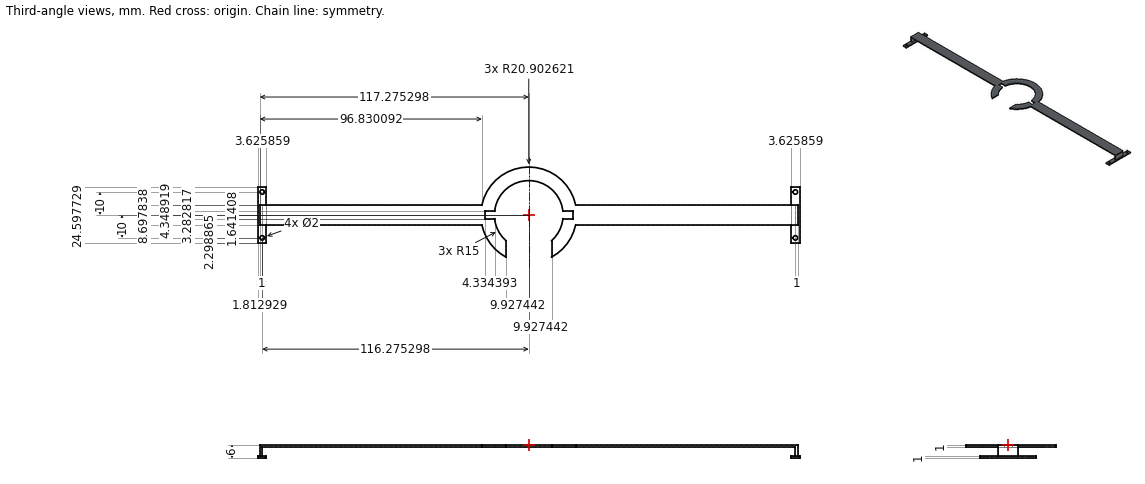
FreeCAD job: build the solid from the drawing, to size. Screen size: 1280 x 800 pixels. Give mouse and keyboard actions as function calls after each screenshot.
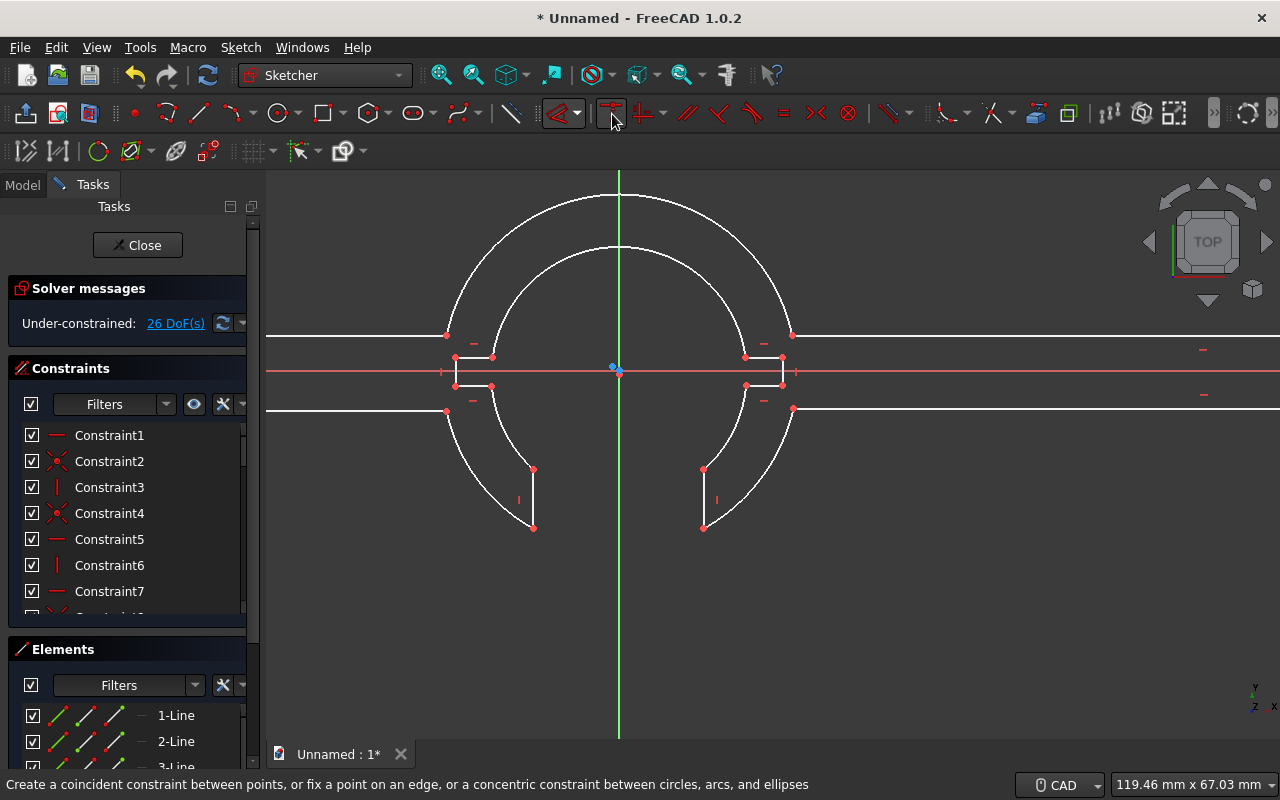
click(462, 454)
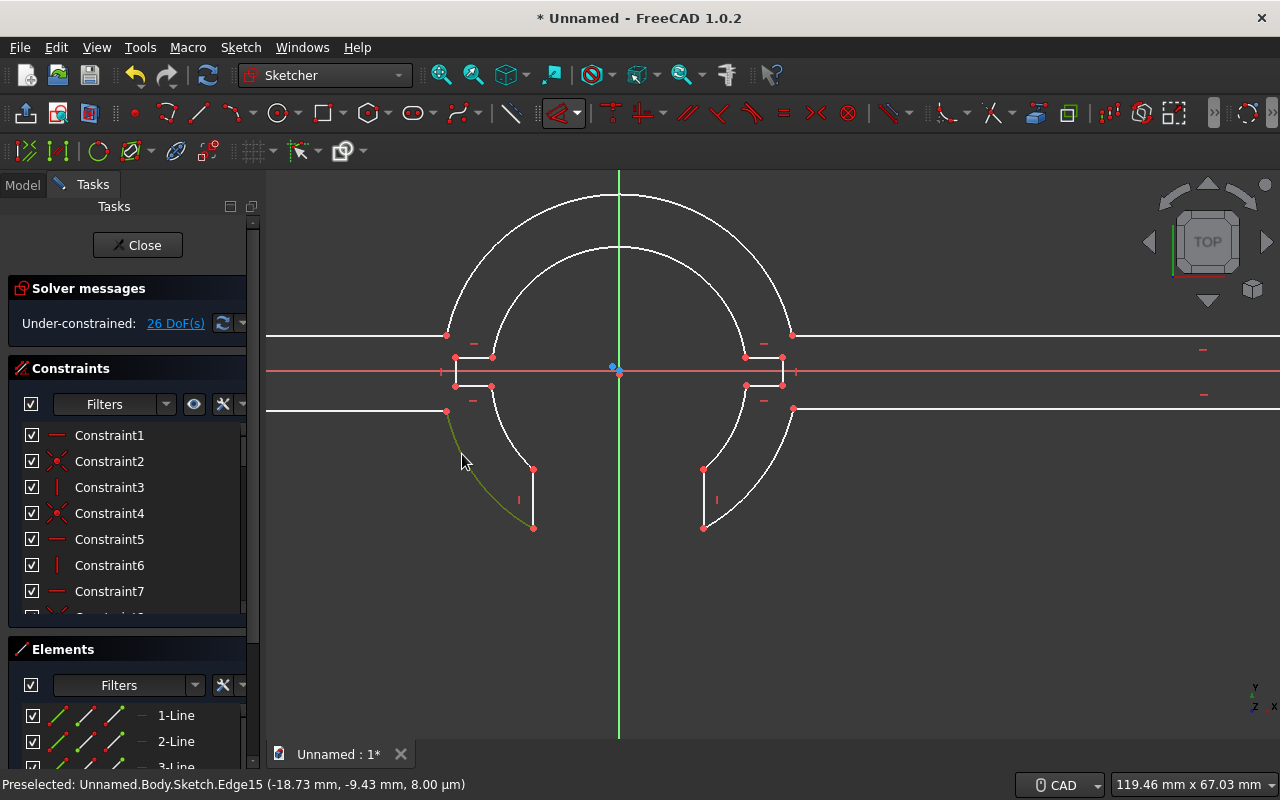
click(741, 501)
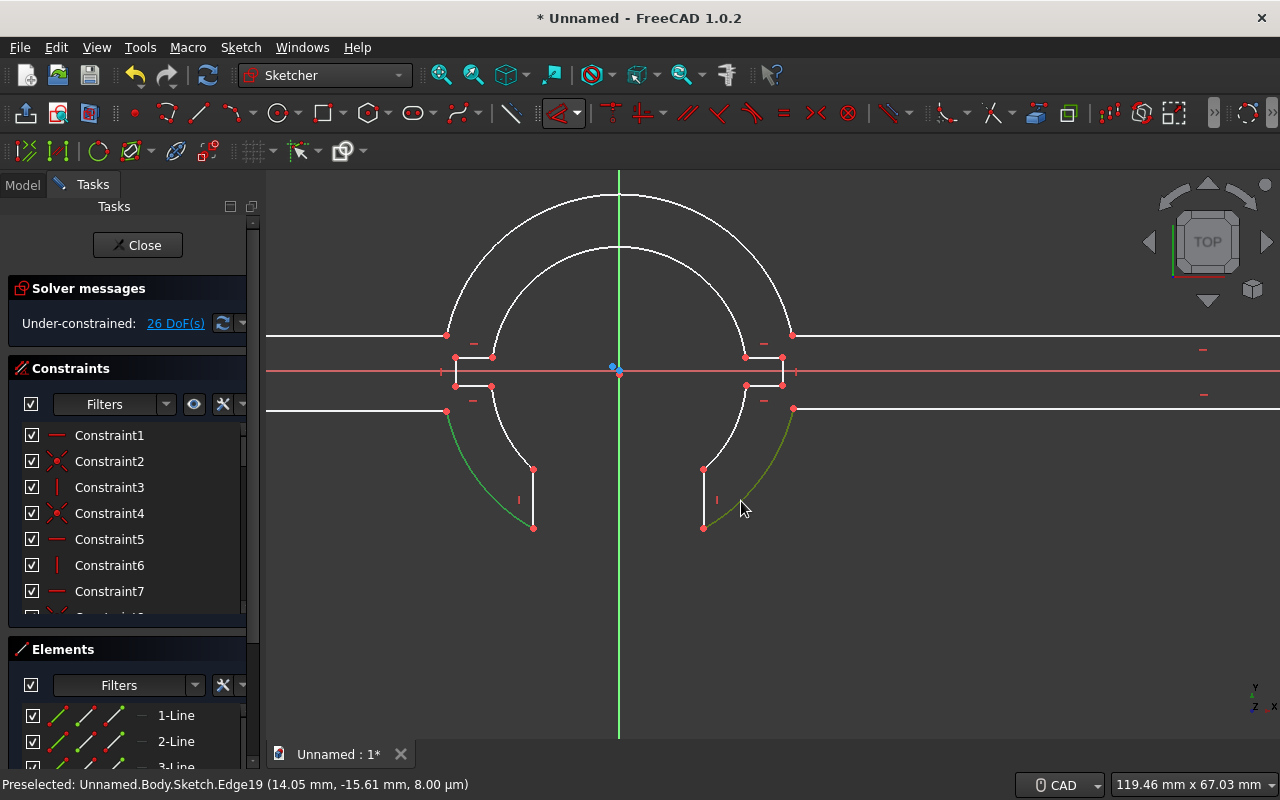
key(c)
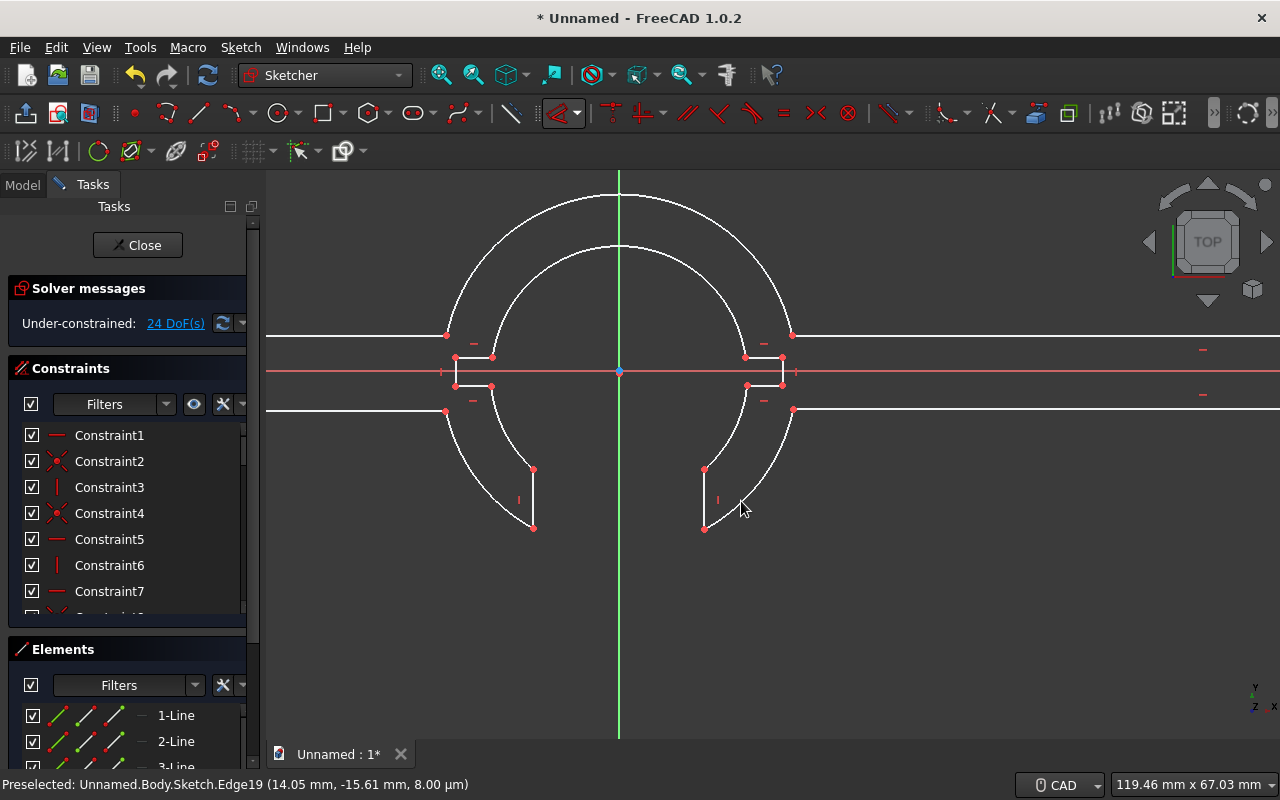
click(461, 454)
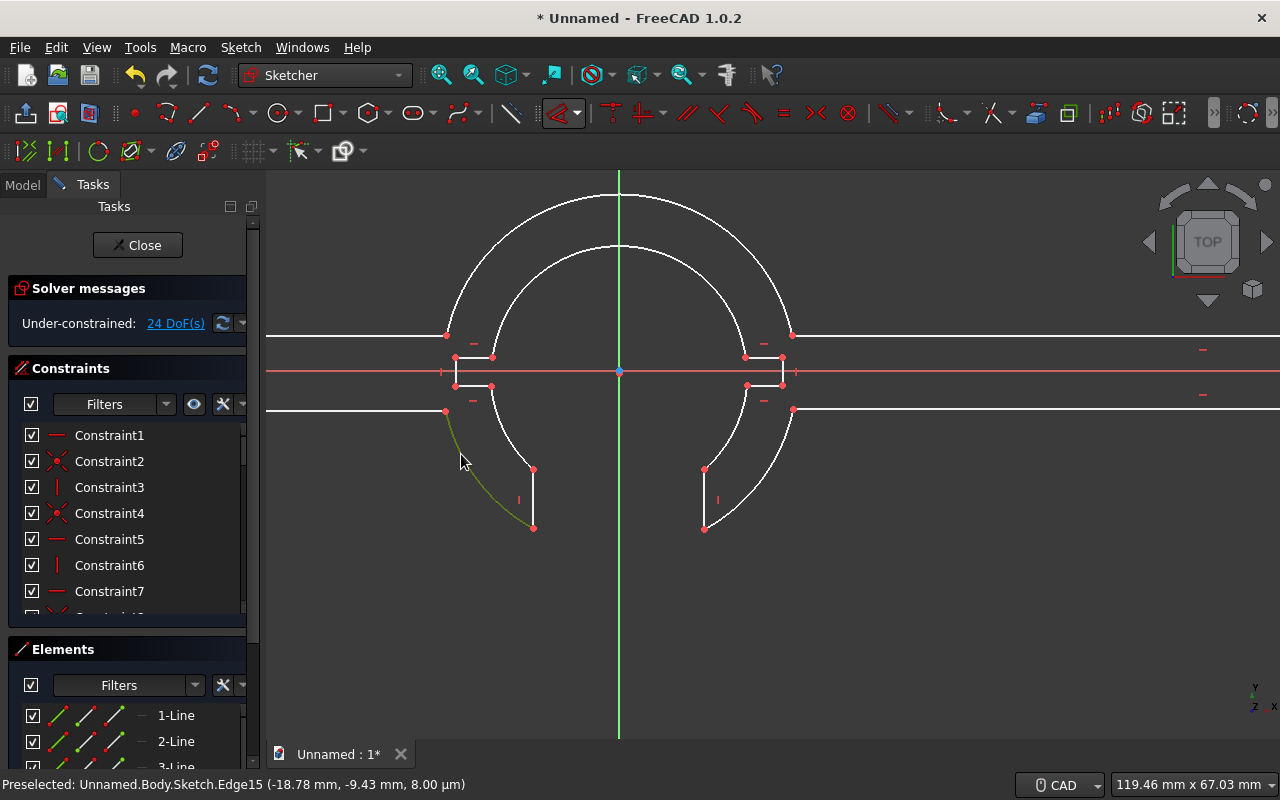
click(711, 220)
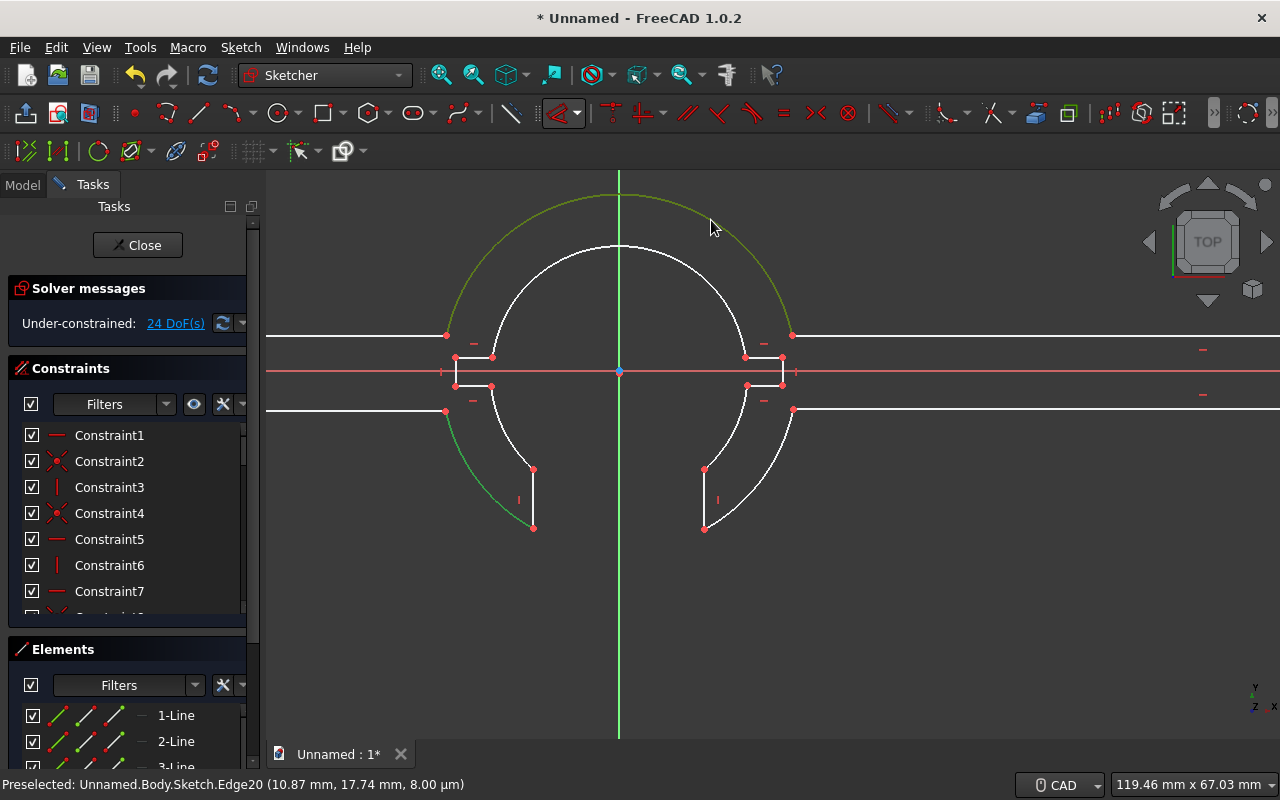
click(612, 114)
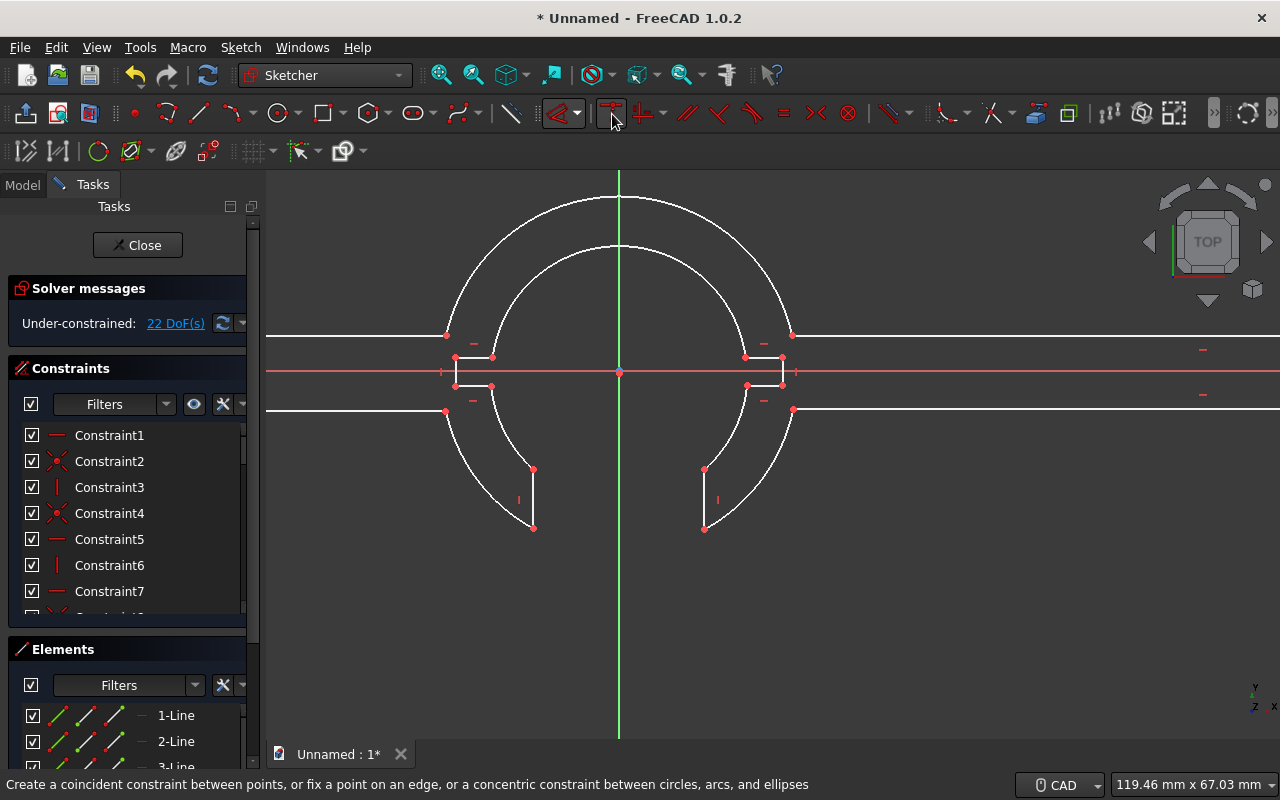
drag(609, 361, 629, 384)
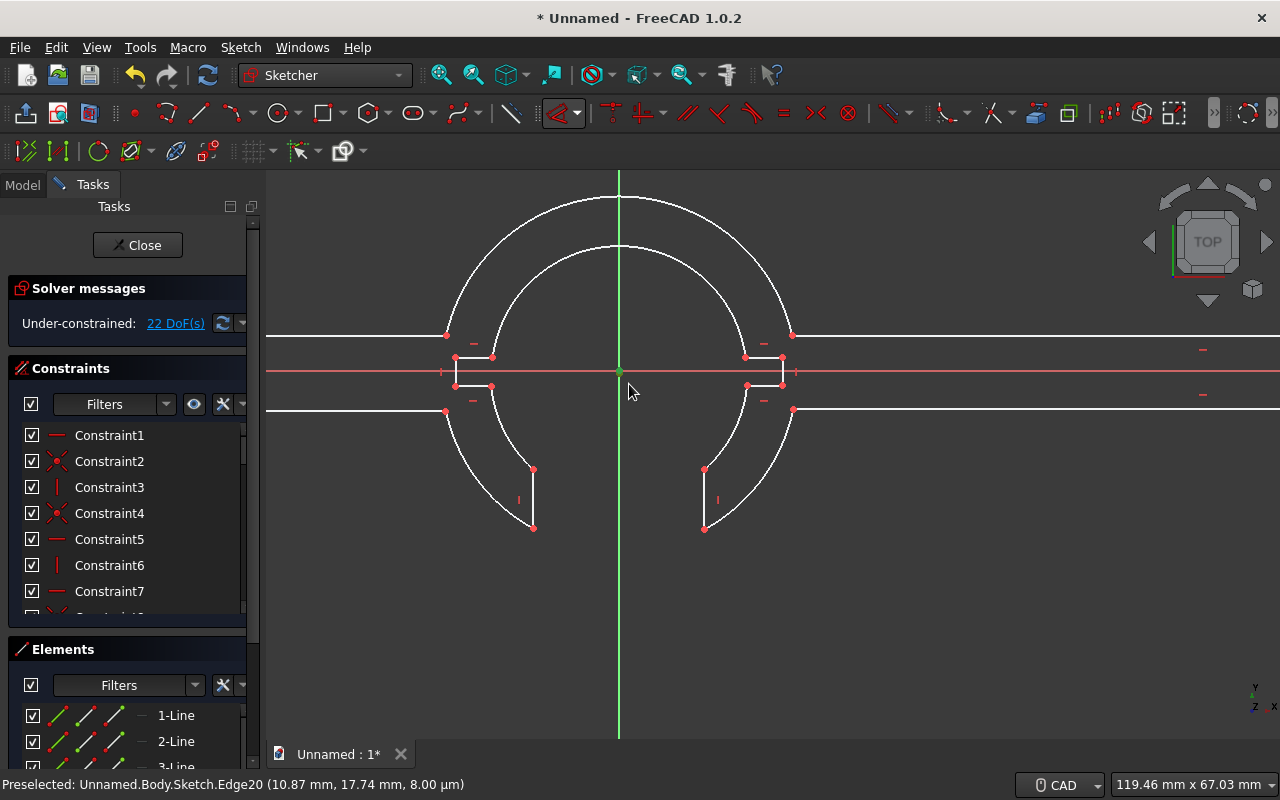
click(612, 114)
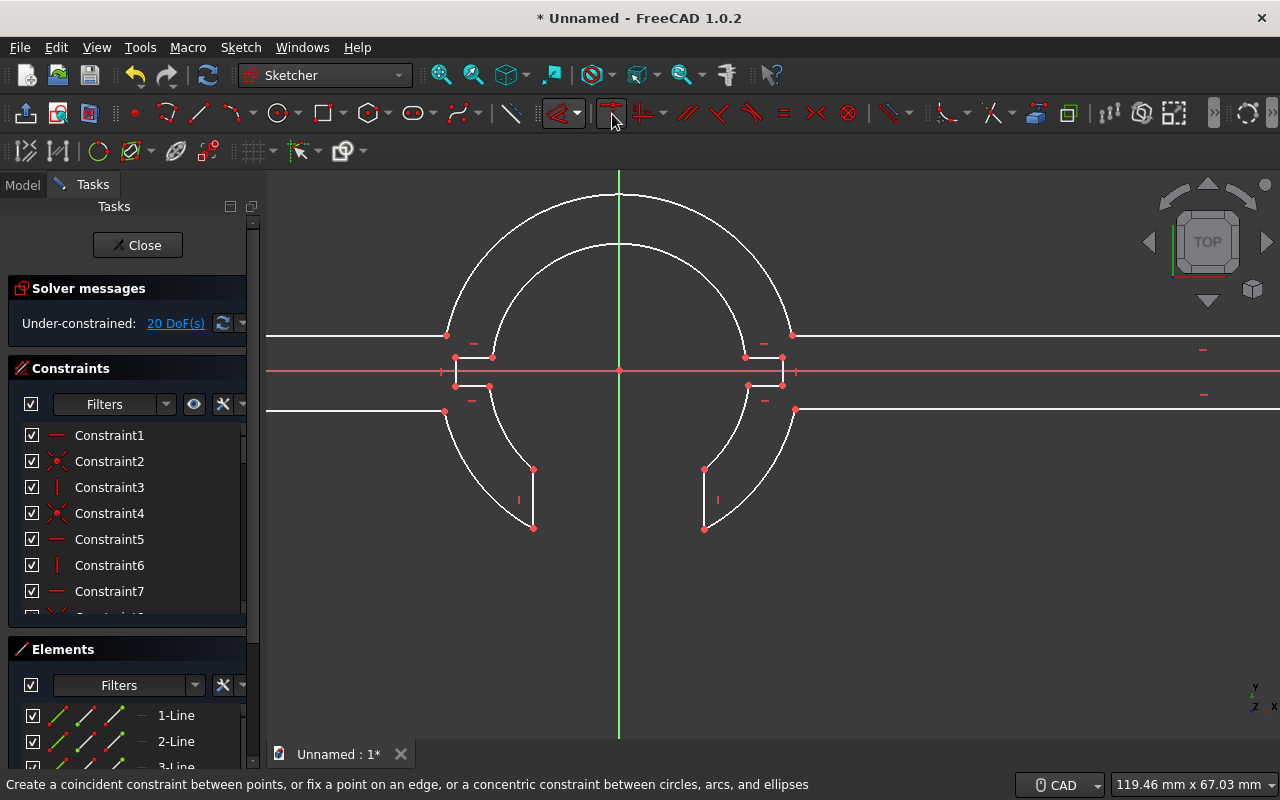
click(496, 414)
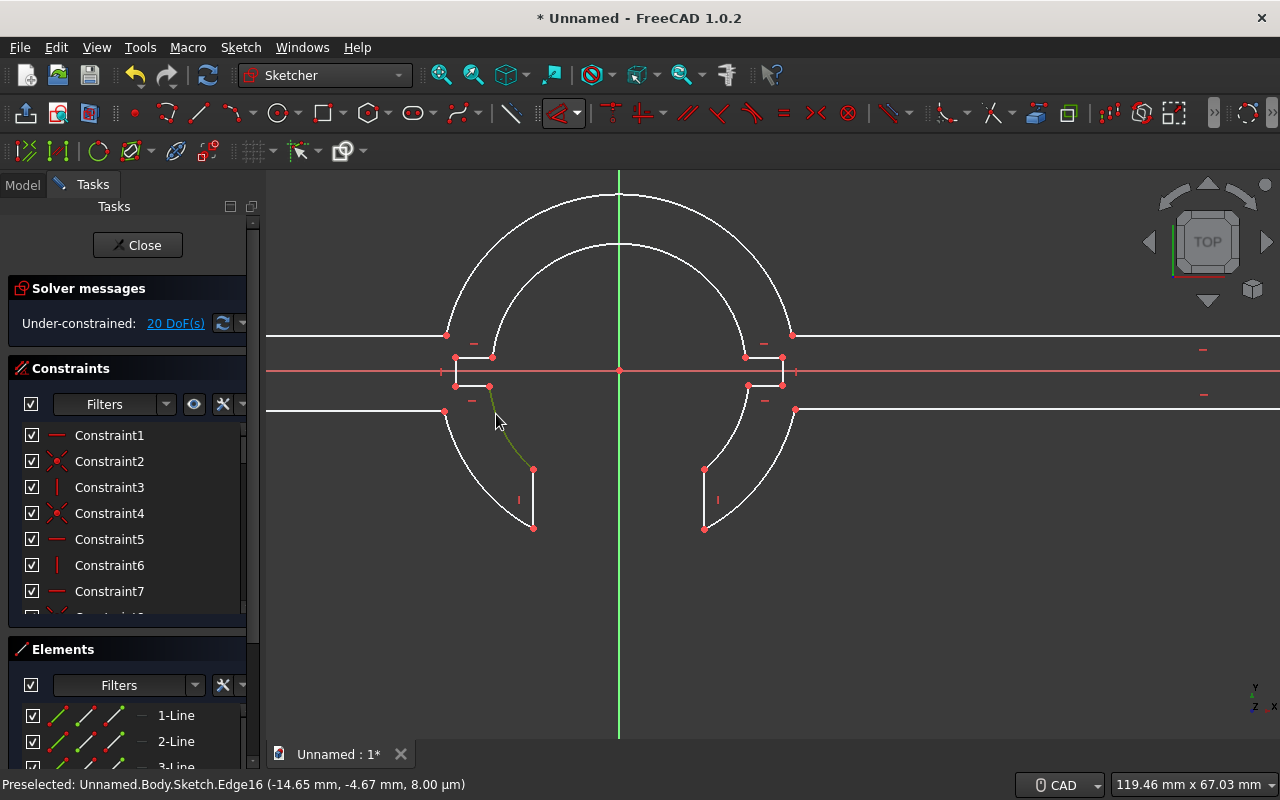
click(689, 265)